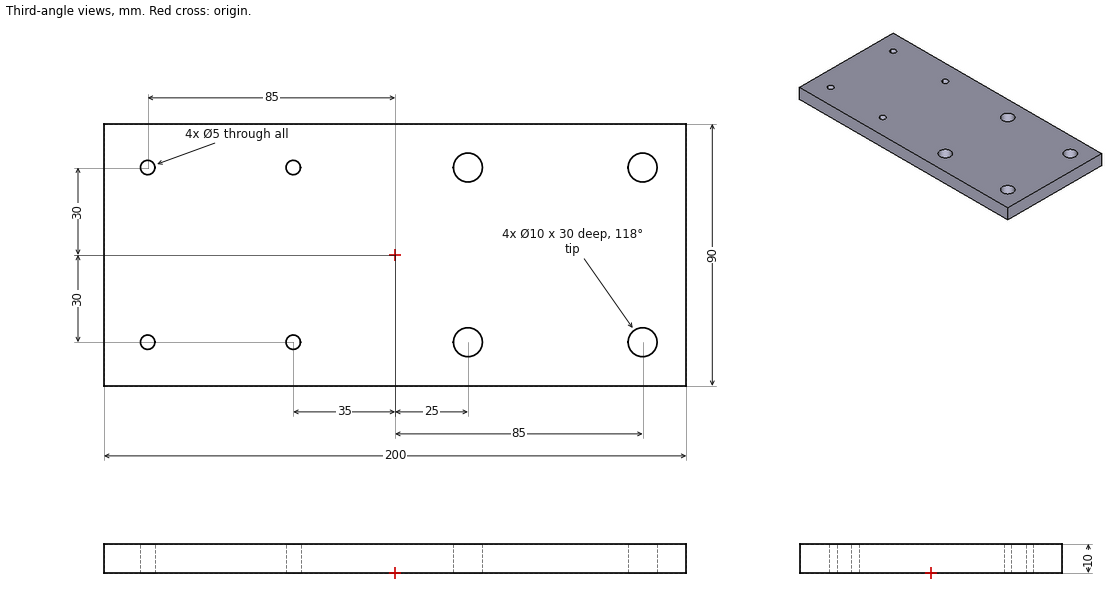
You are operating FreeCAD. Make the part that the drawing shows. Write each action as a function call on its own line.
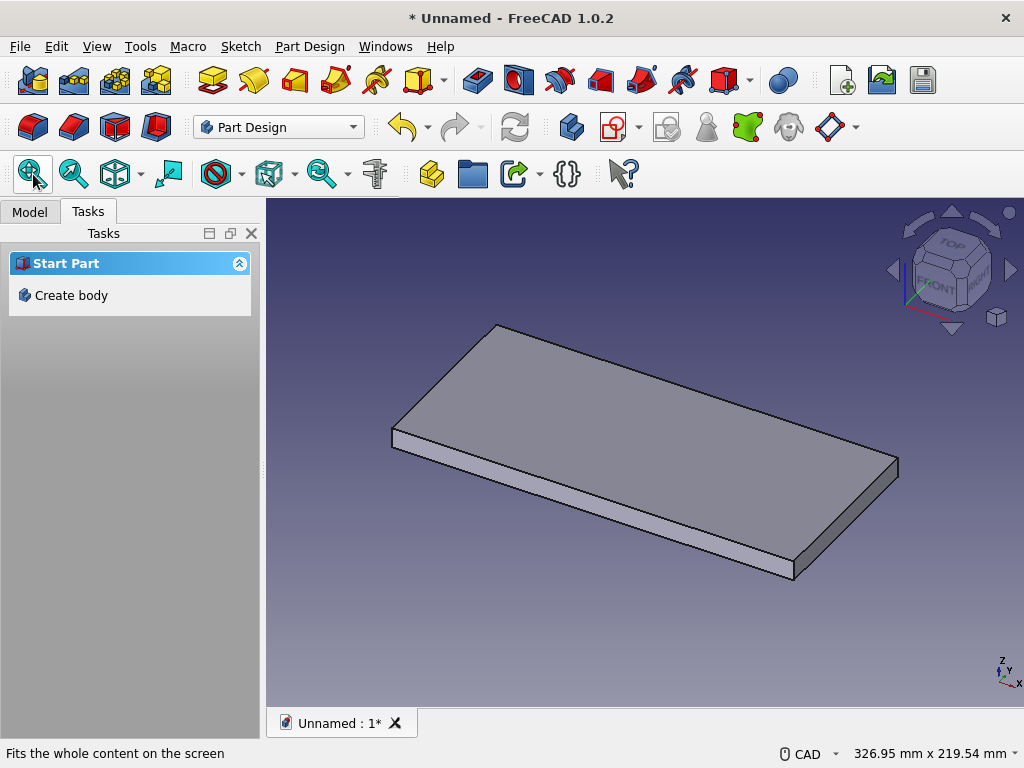
click(612, 128)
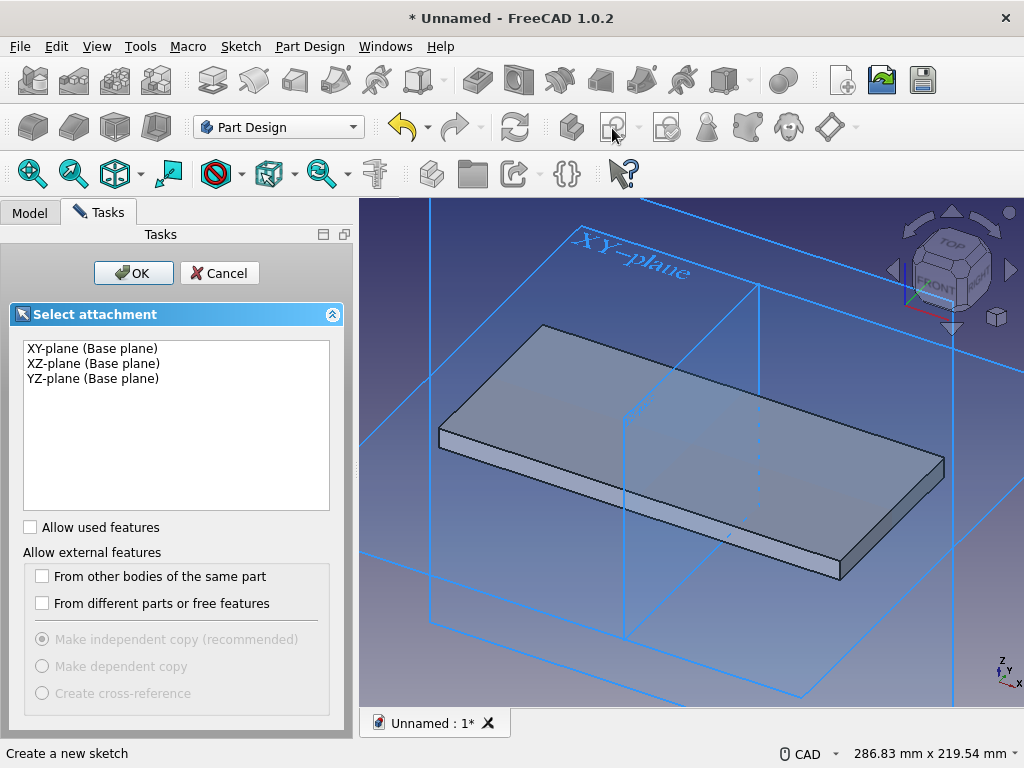
click(84, 348)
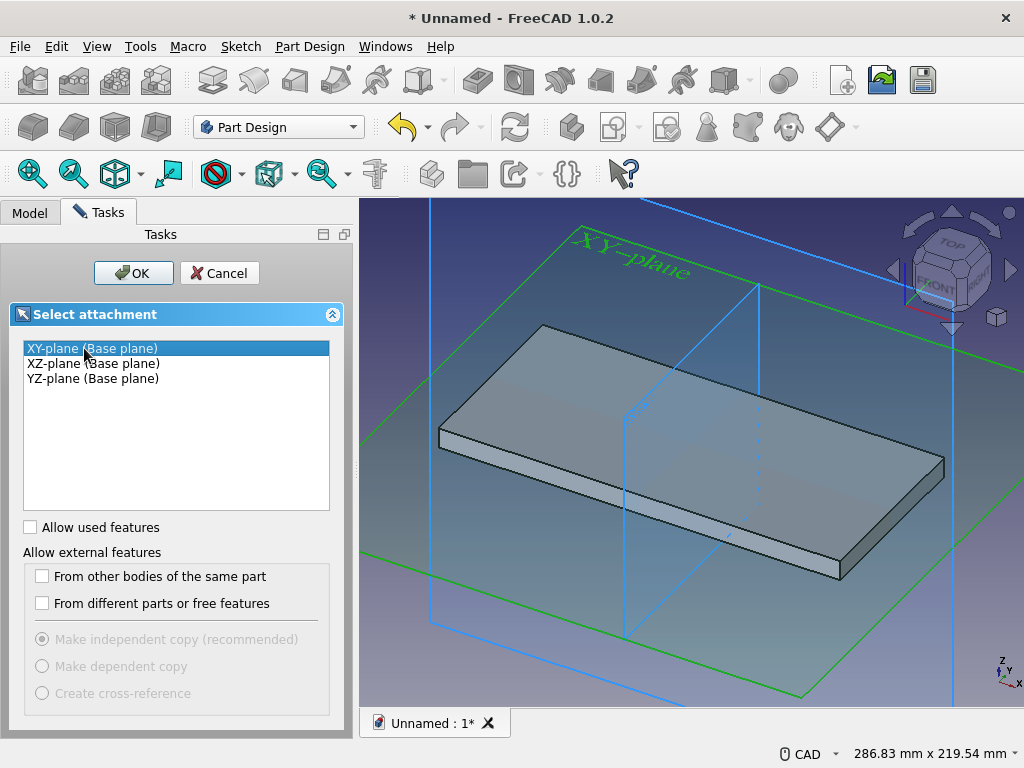
click(134, 273)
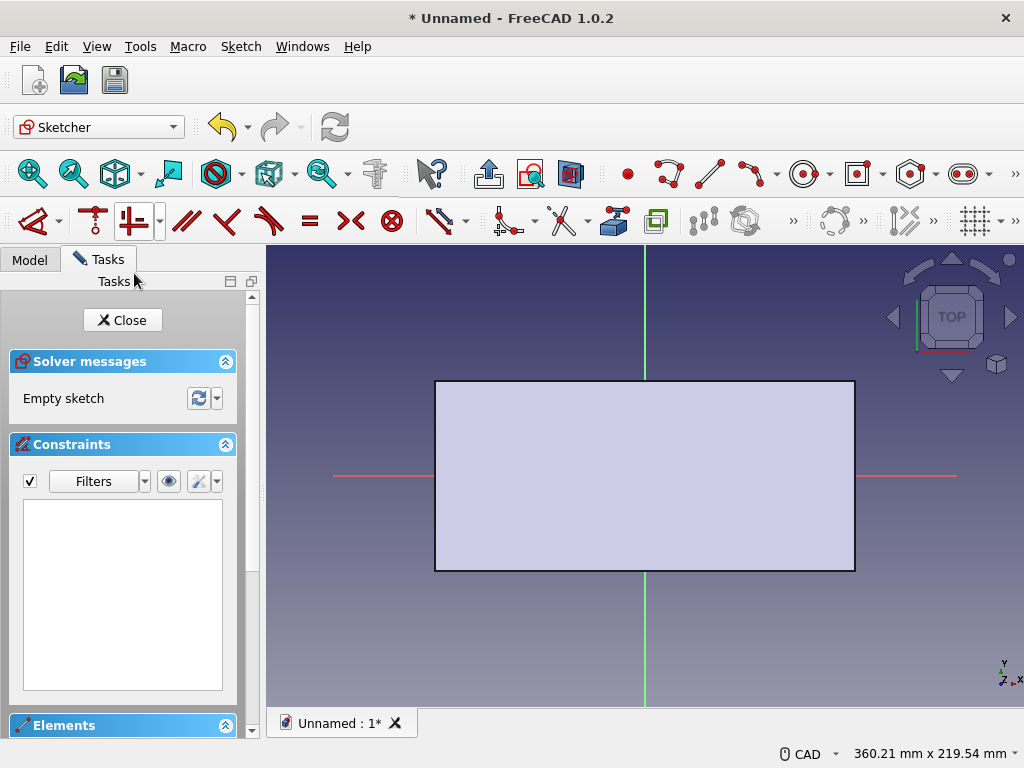
key(q)
key(s)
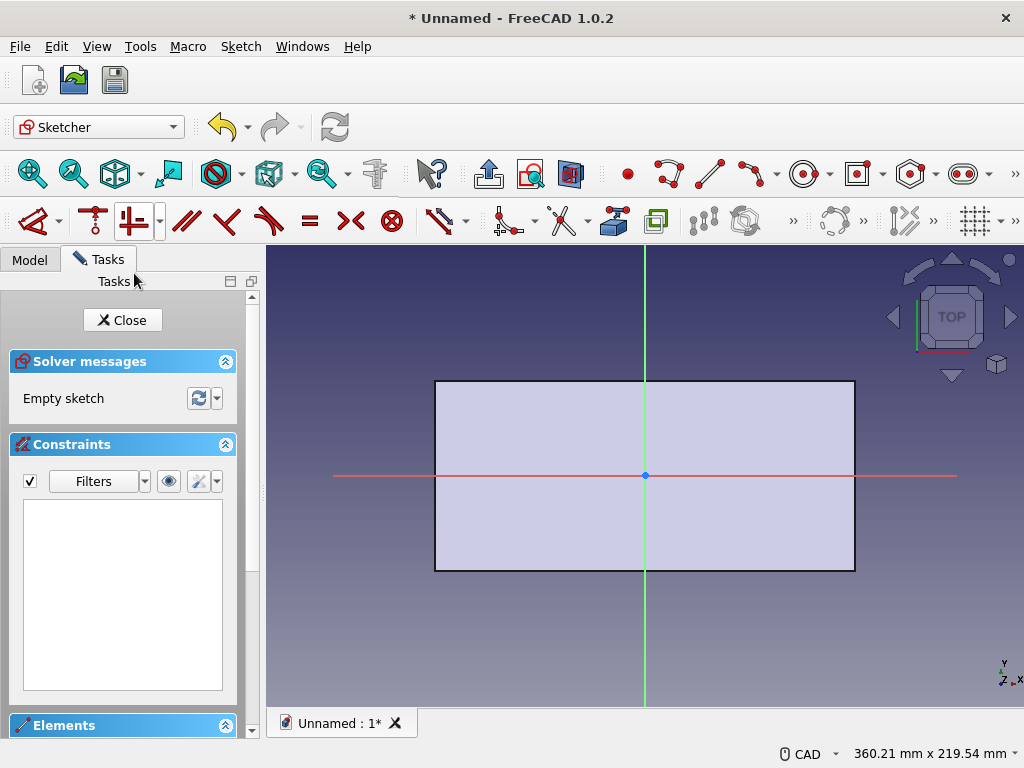
scroll(534, 476, up, 4)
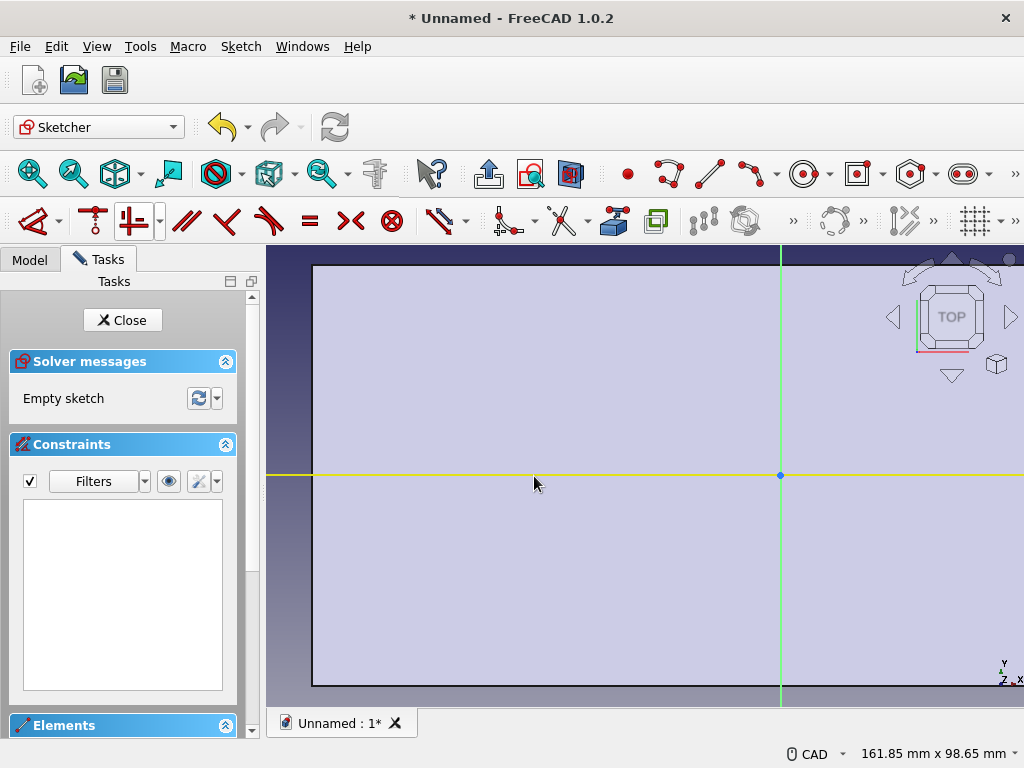
key(g)
key(c)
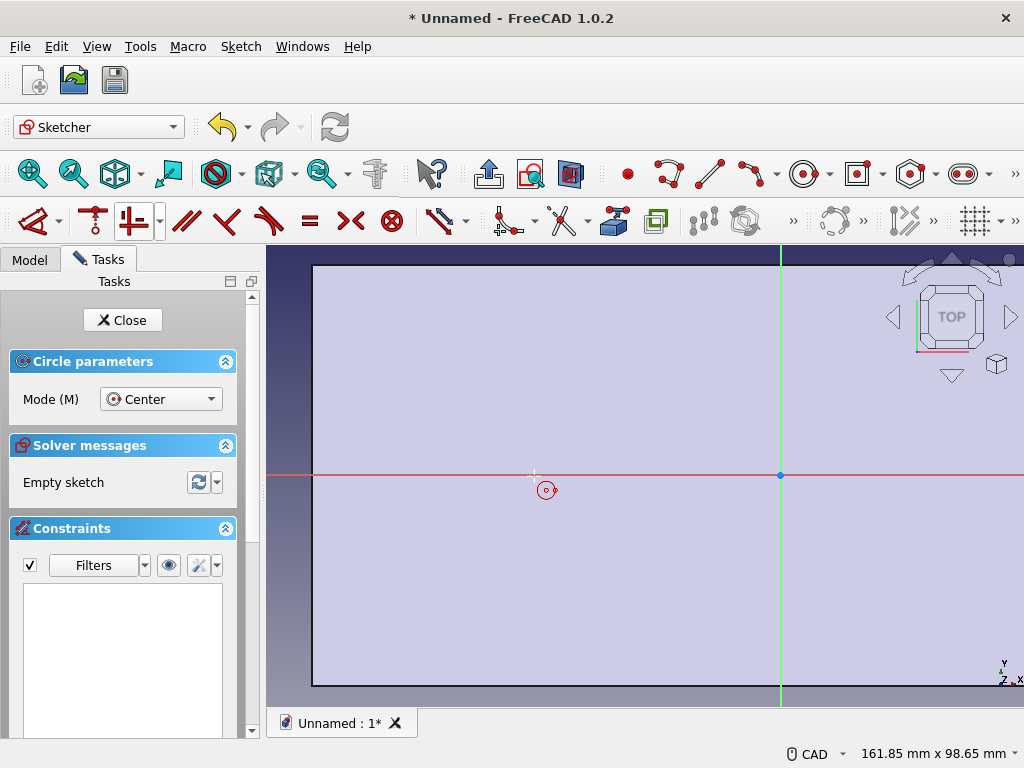
scroll(383, 335, up, 4)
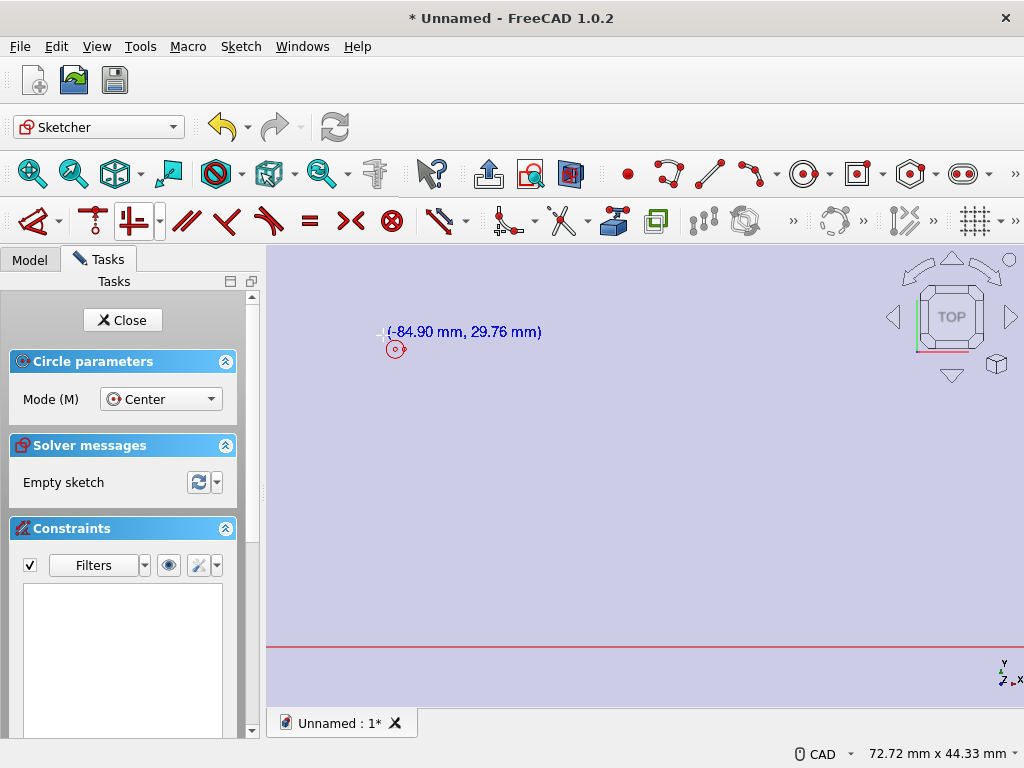
click(382, 335)
move(400, 316)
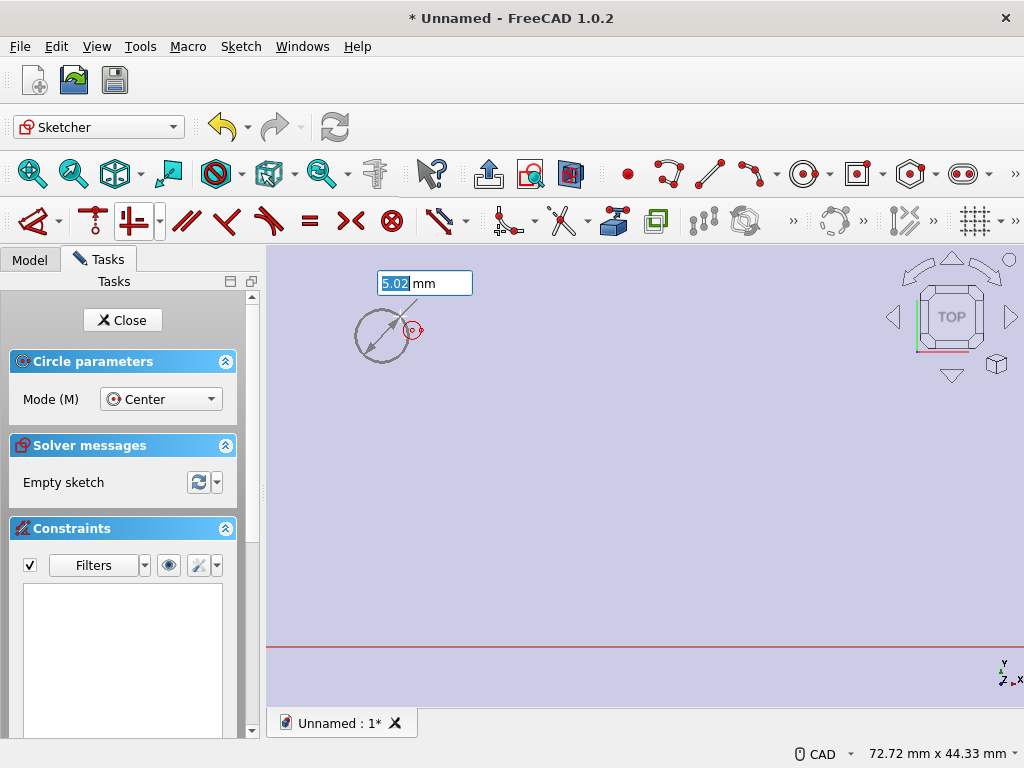
text(5)
key(Return)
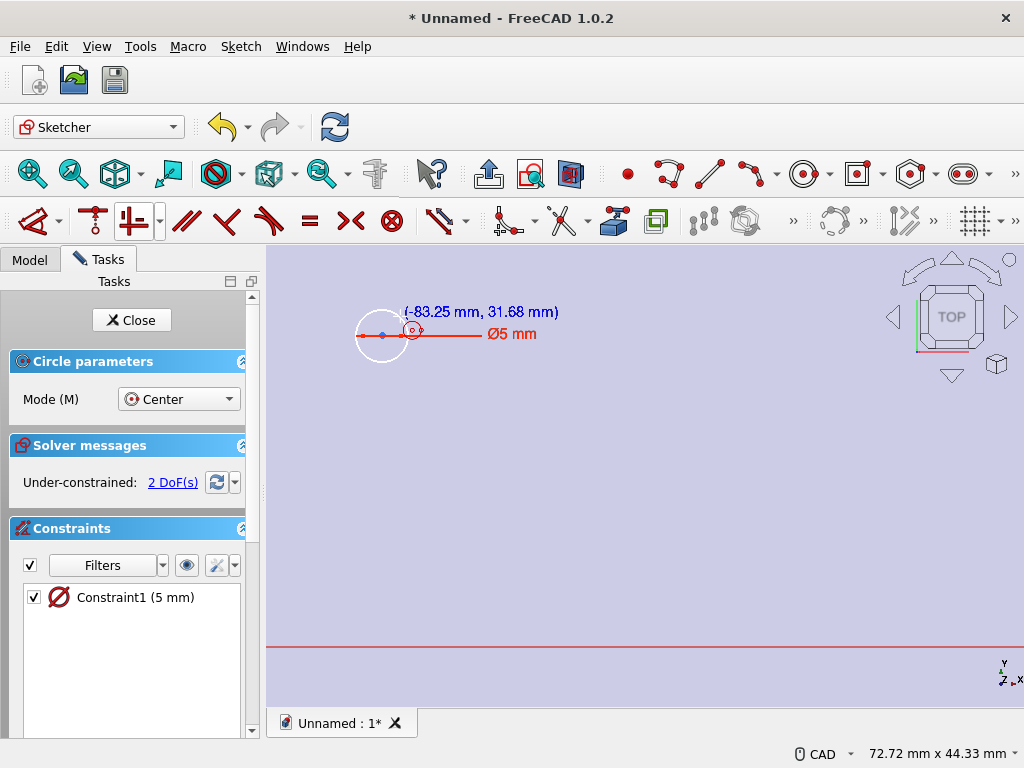
scroll(385, 336, down, 4)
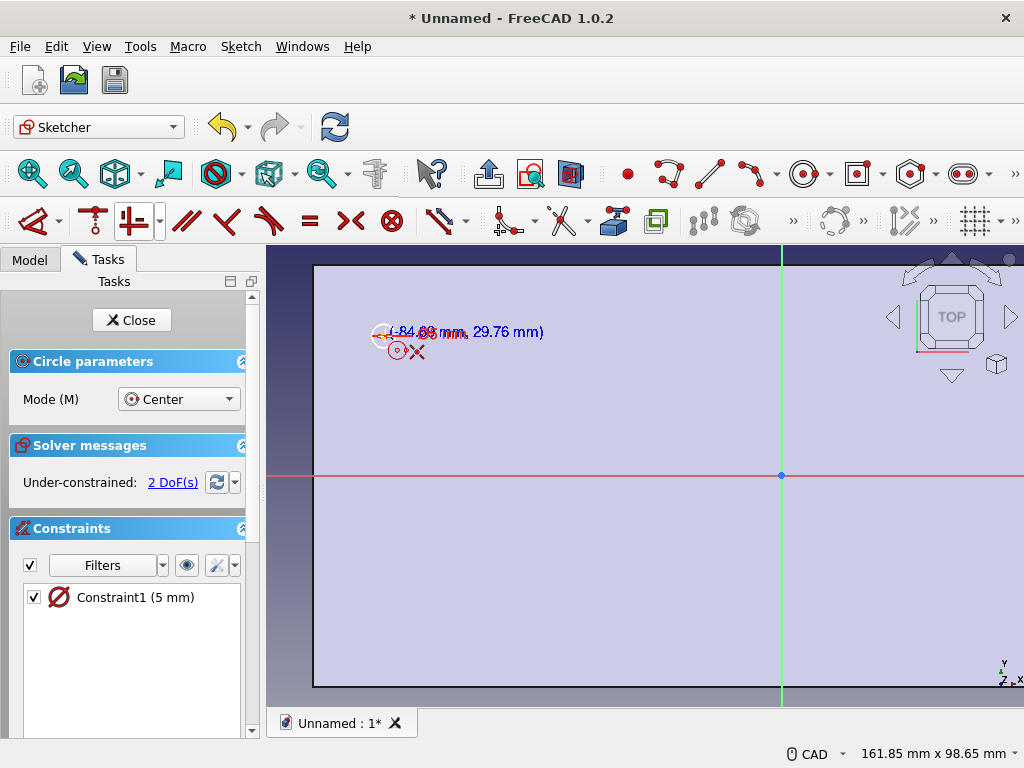
scroll(618, 616, up, 4)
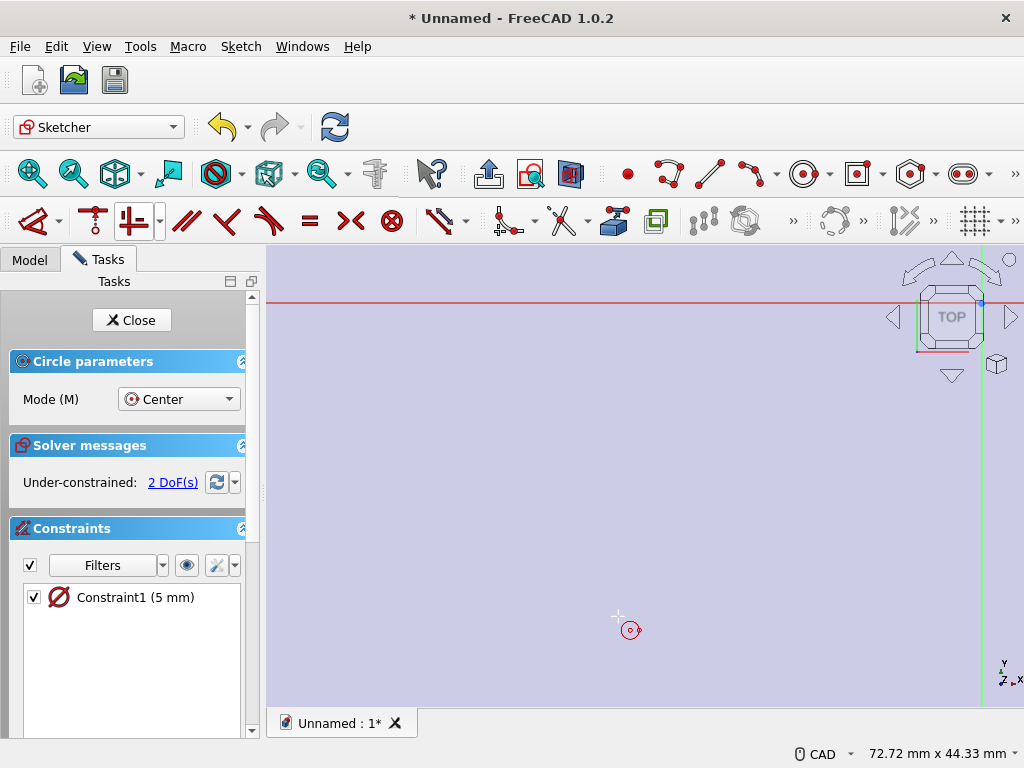
click(617, 616)
move(635, 598)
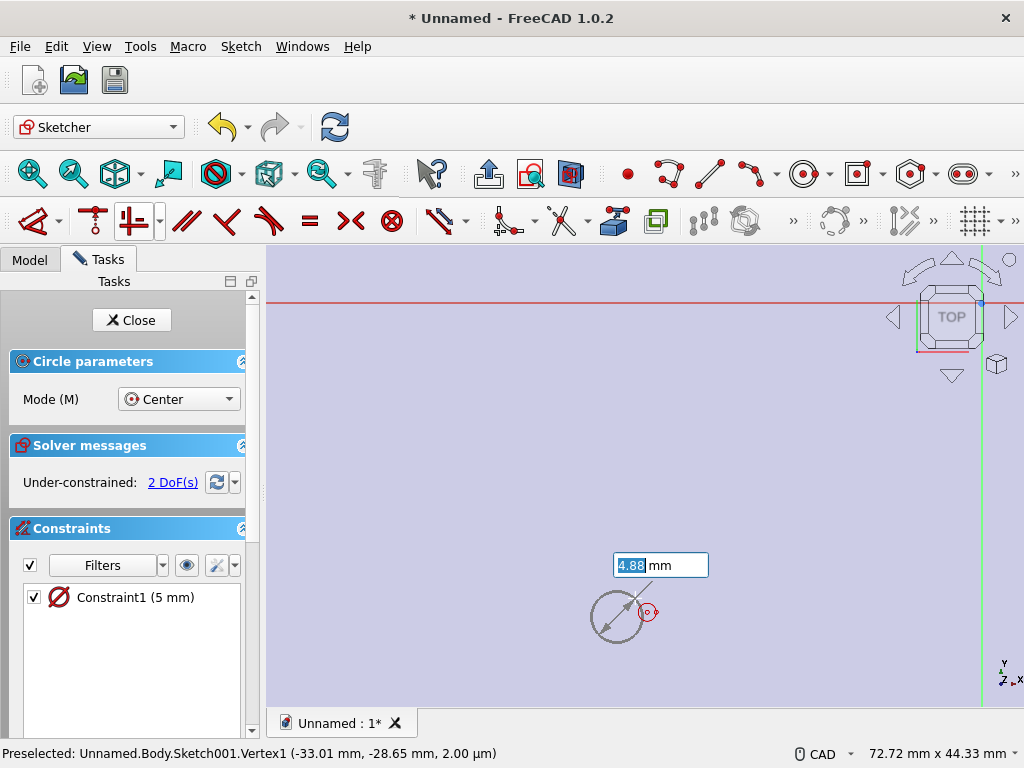
text(5)
key(Return)